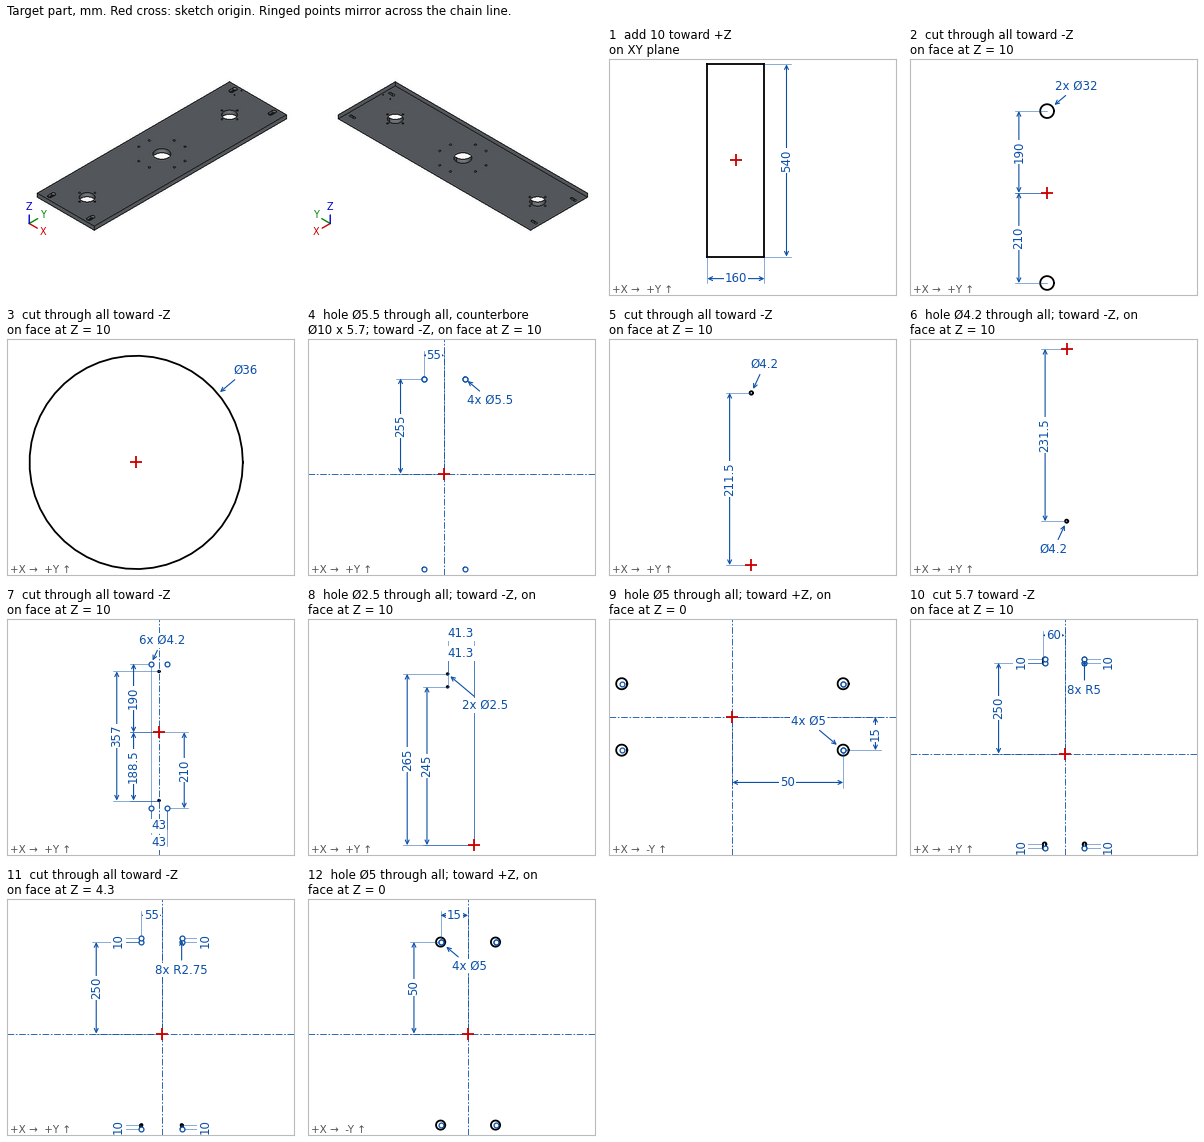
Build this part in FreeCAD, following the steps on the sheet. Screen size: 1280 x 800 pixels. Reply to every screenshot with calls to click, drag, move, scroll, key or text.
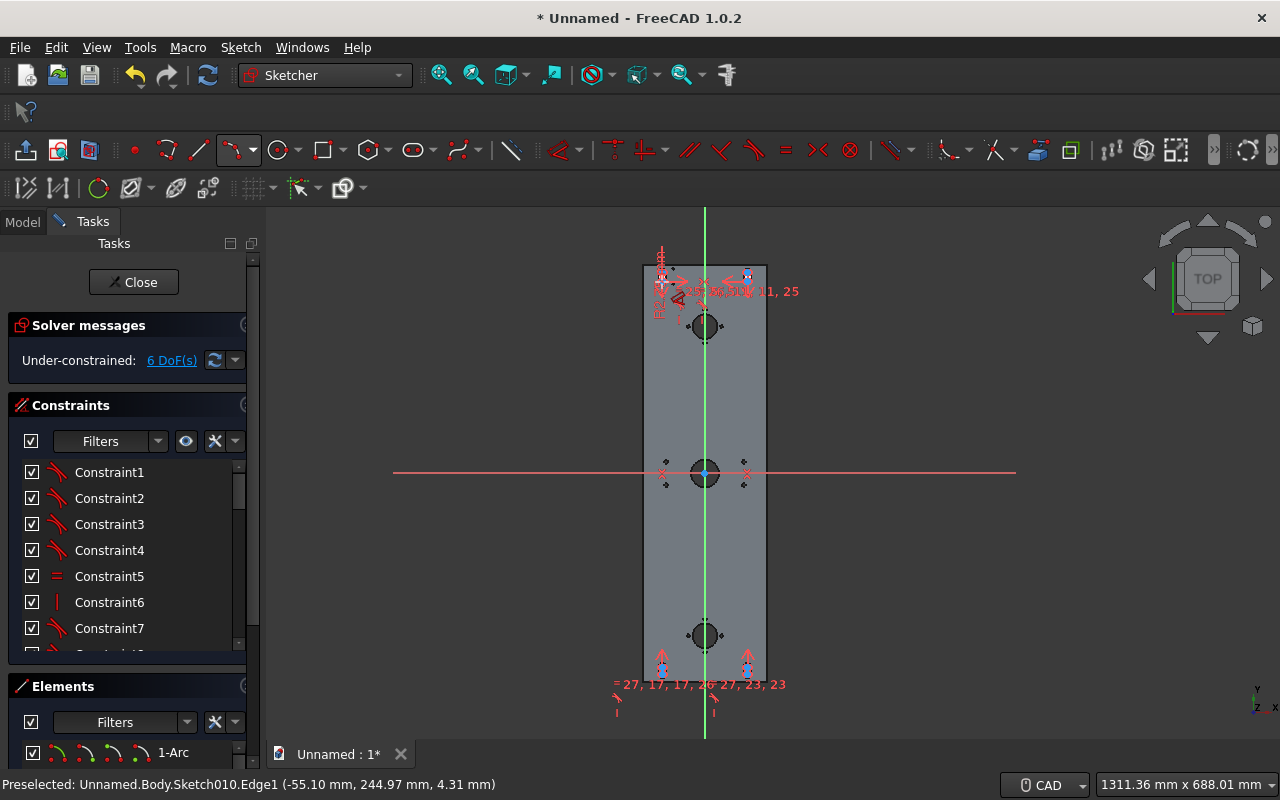
scroll(660, 279, up, 9)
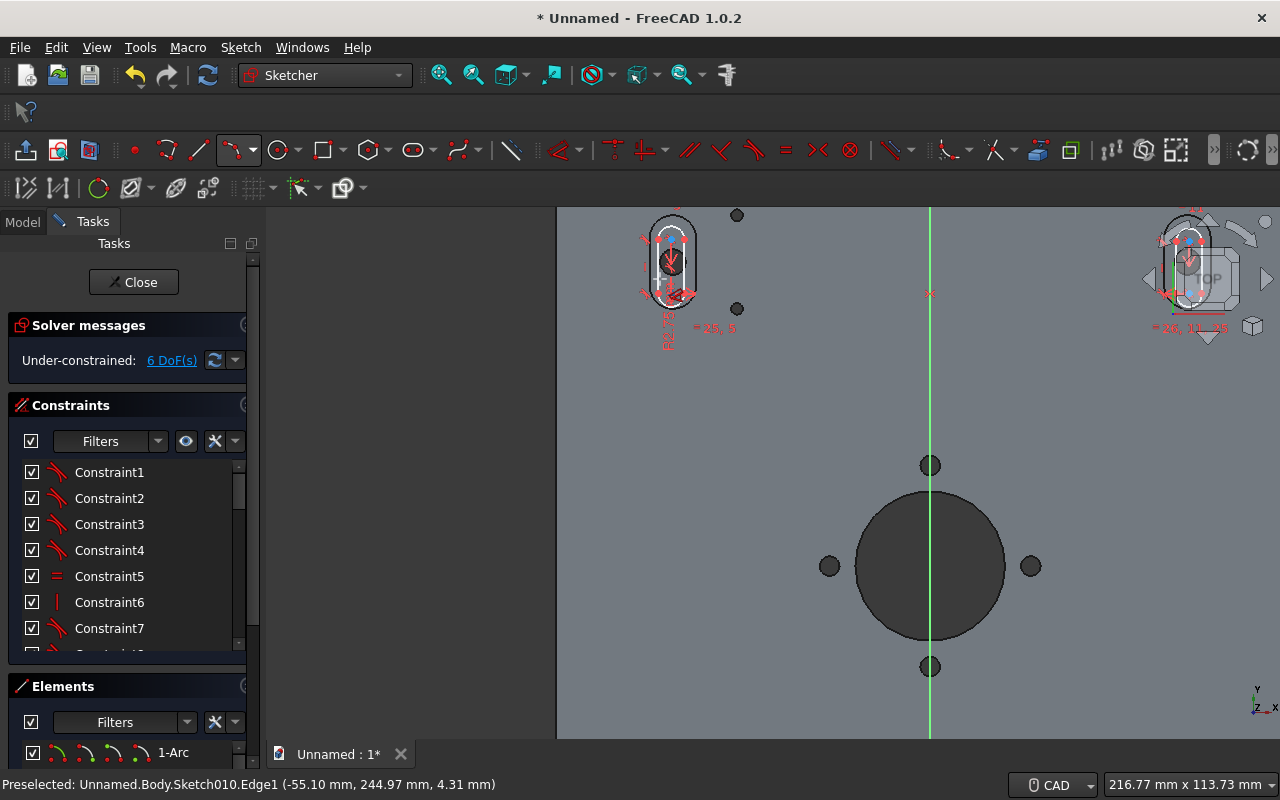
click(658, 278)
click(624, 267)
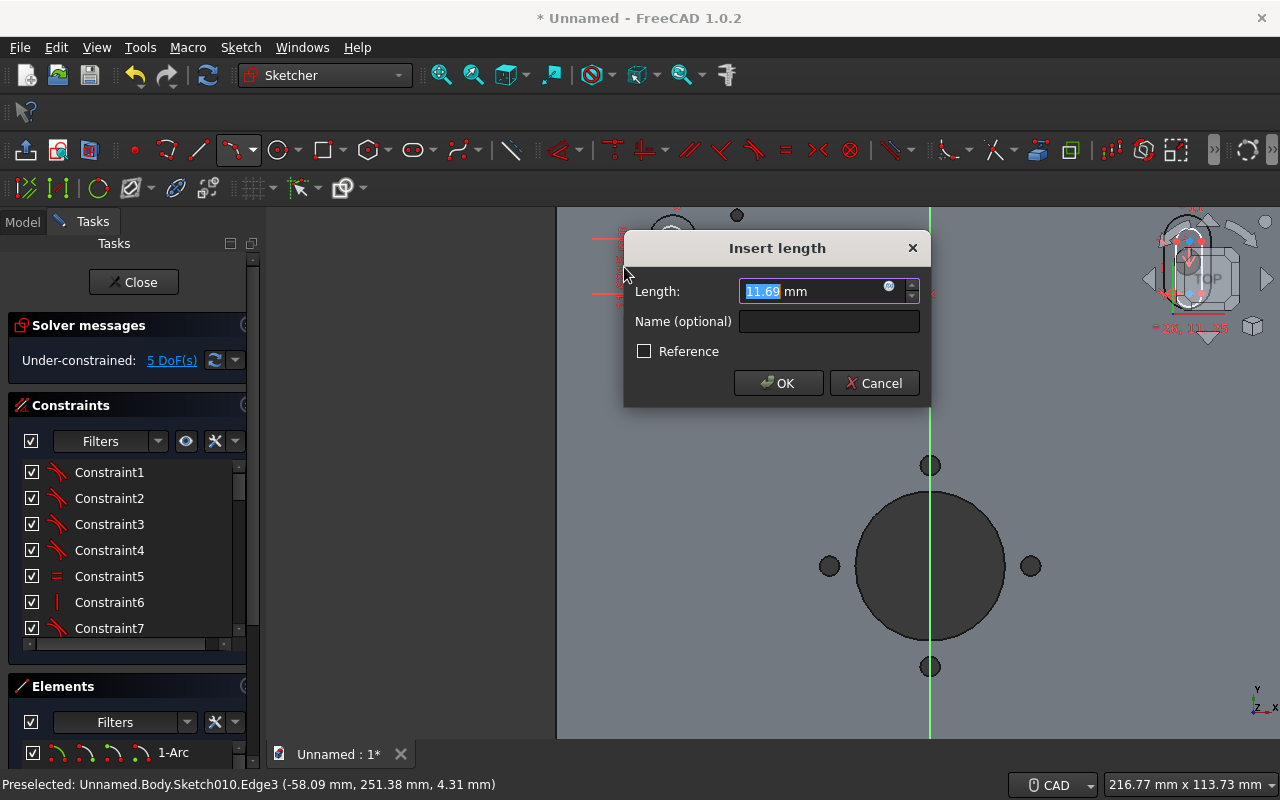
text(10)
key(Return)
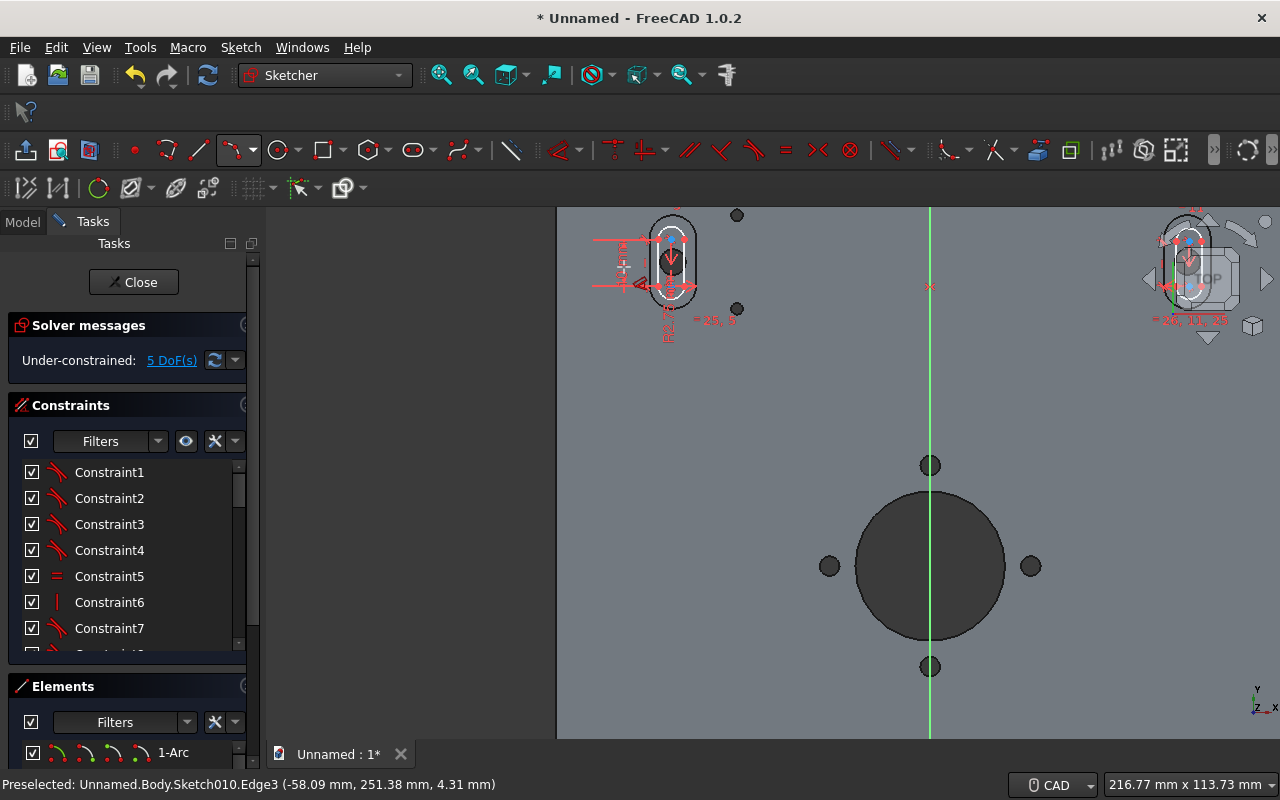
scroll(669, 319, down, 10)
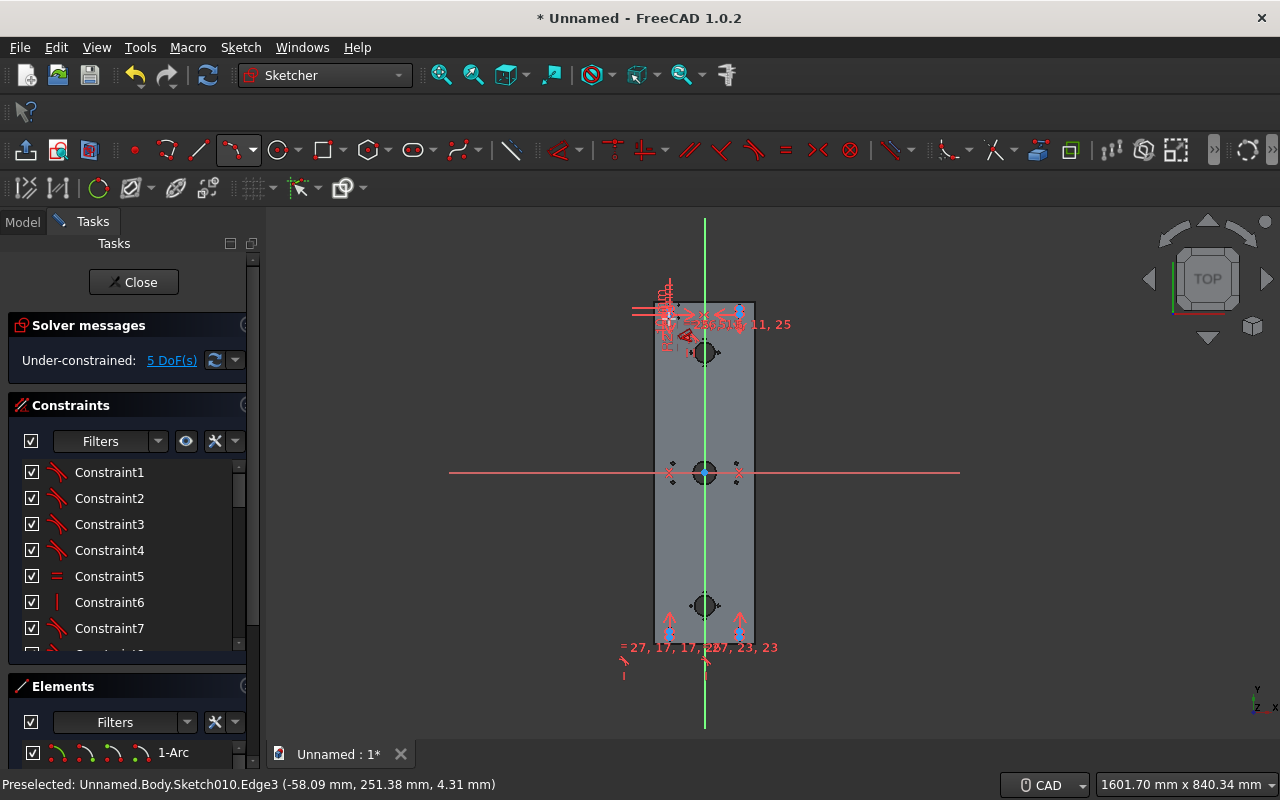
scroll(738, 313, up, 11)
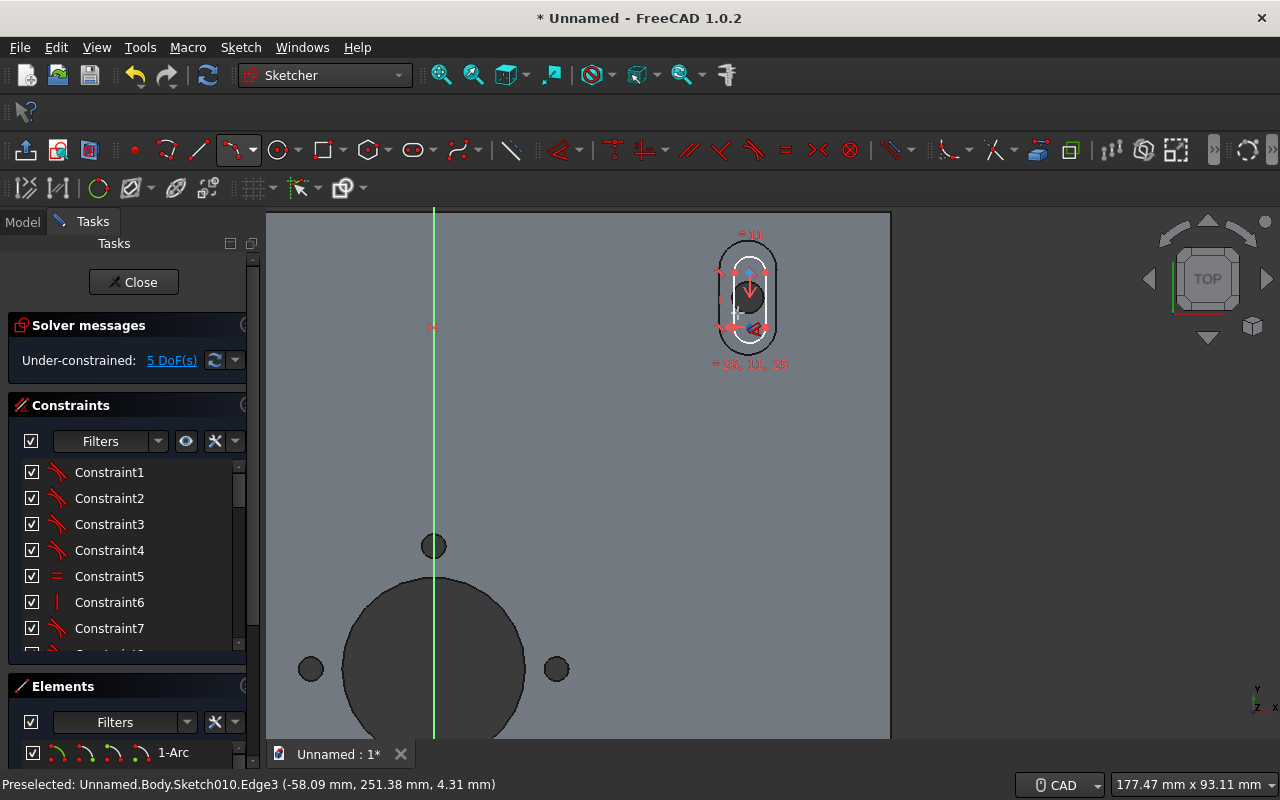
click(734, 311)
click(700, 300)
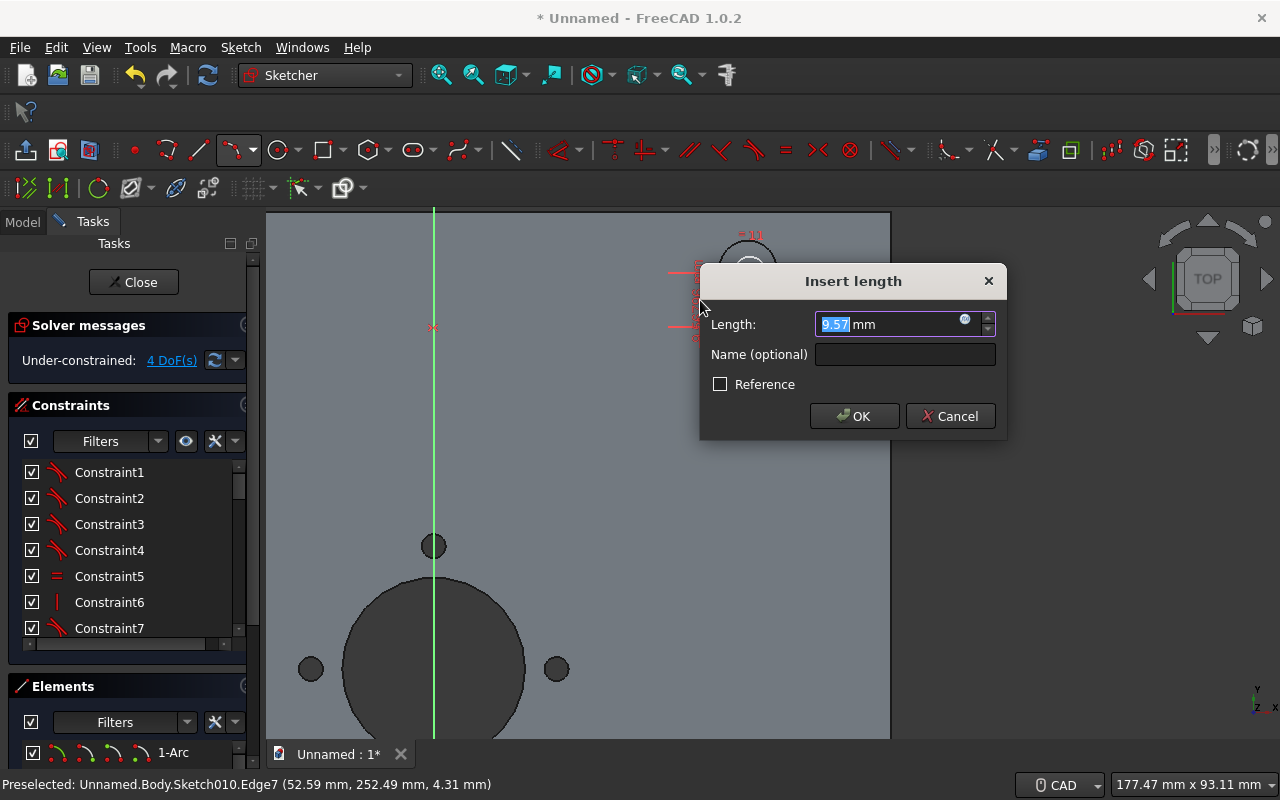
text(10)
key(Return)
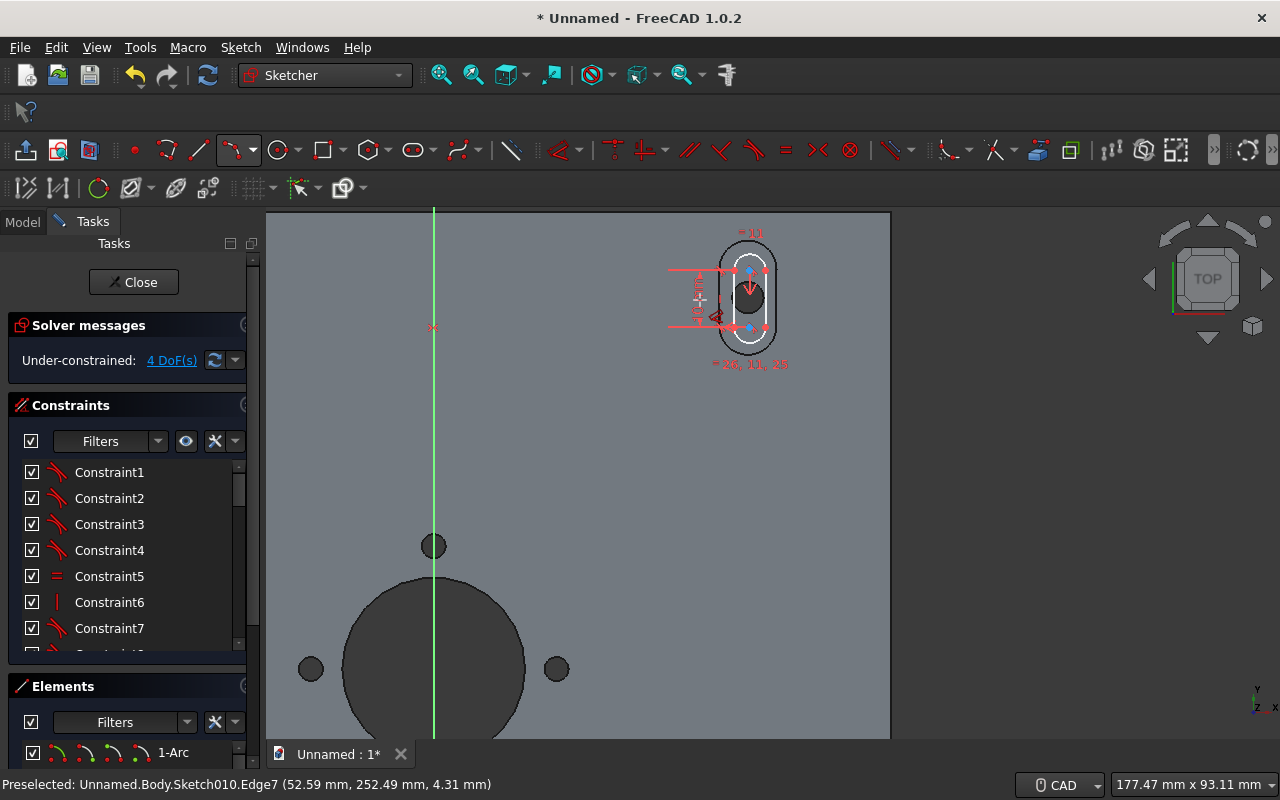
scroll(738, 313, down, 11)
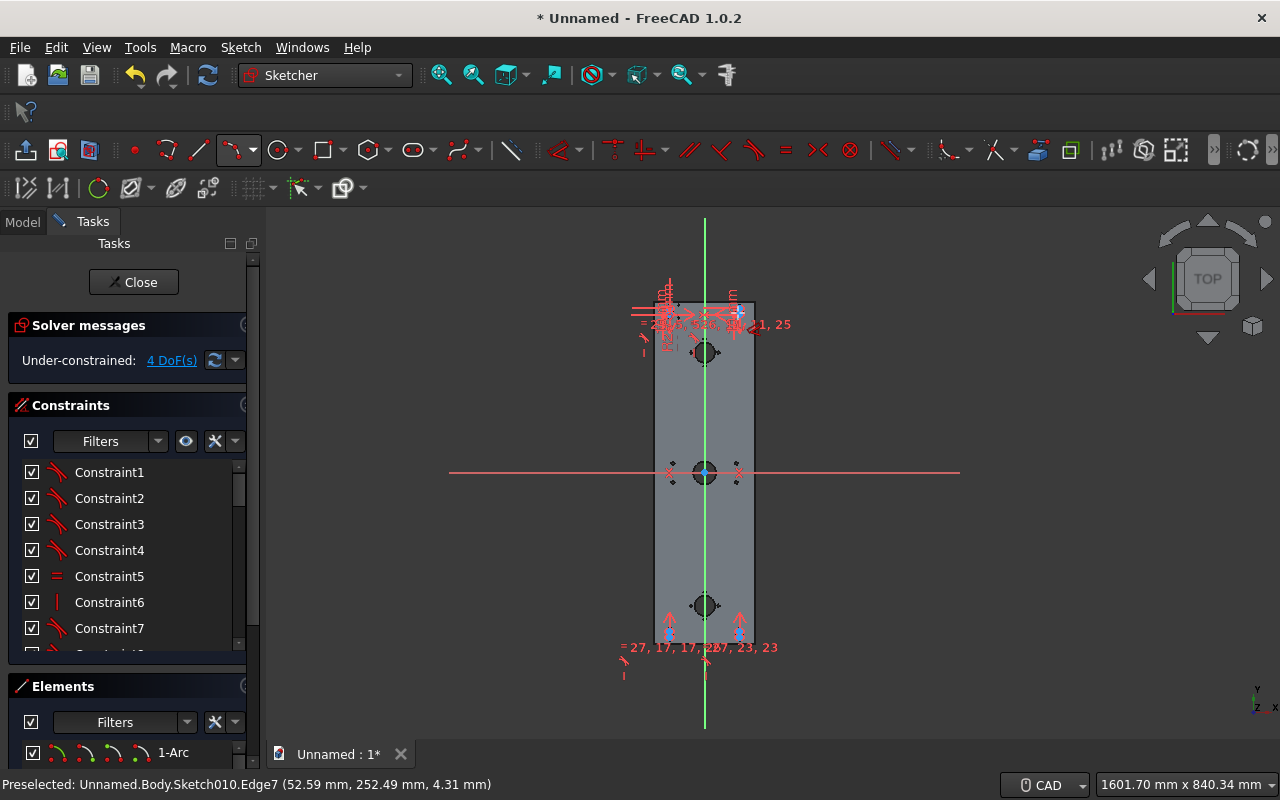
scroll(668, 636, up, 11)